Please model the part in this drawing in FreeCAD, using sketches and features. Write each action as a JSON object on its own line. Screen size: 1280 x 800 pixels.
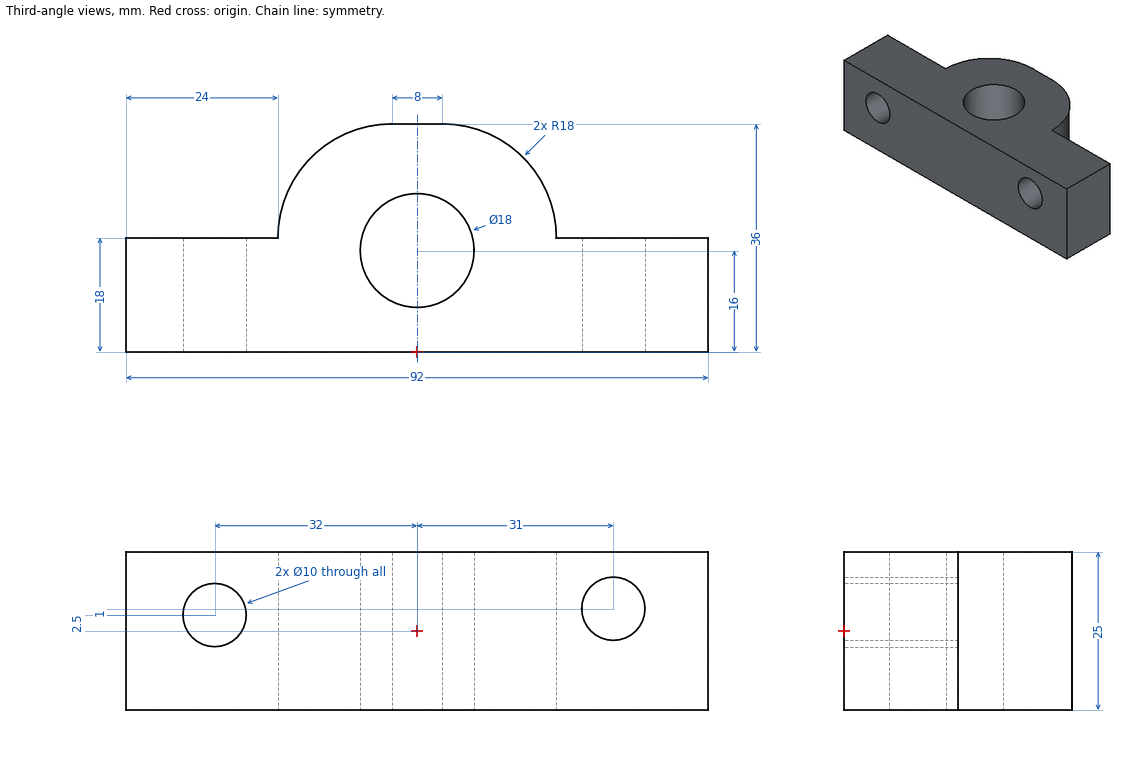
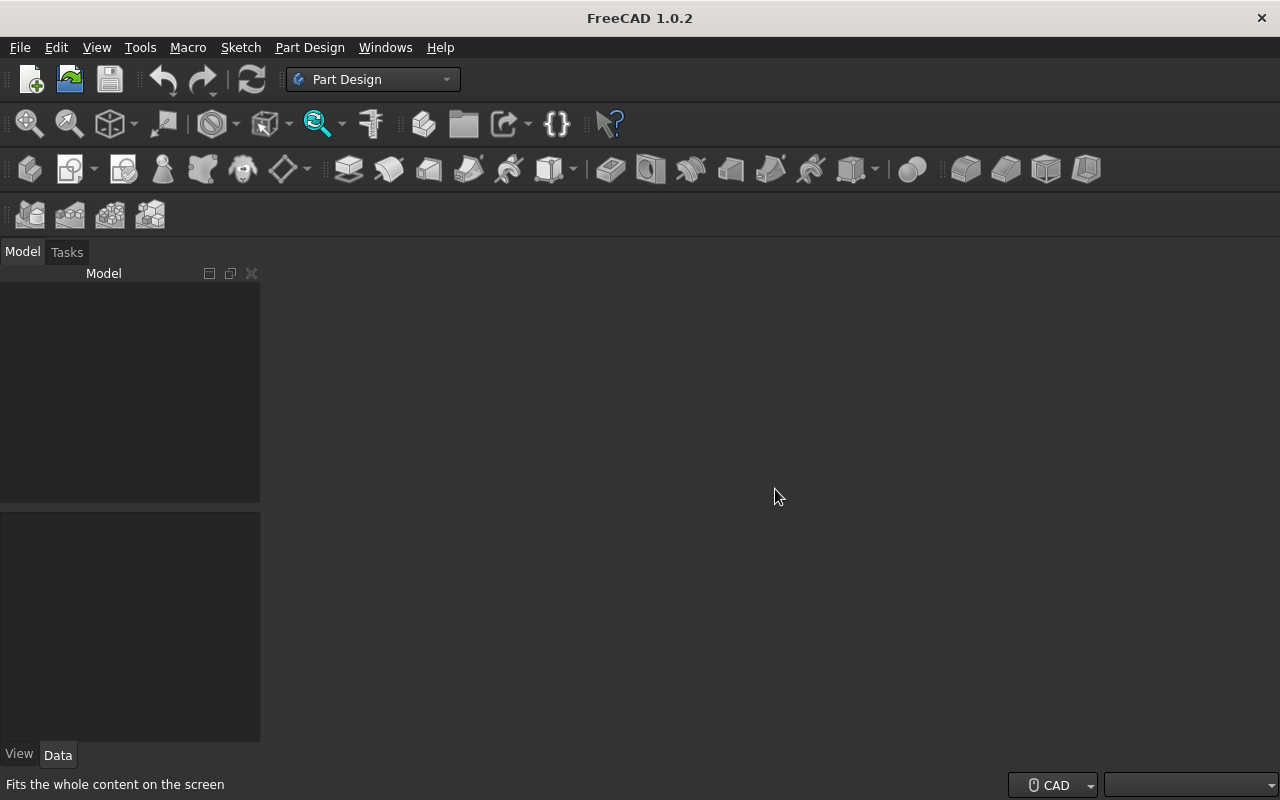
{"action": "left_click", "coordinate": [30, 80]}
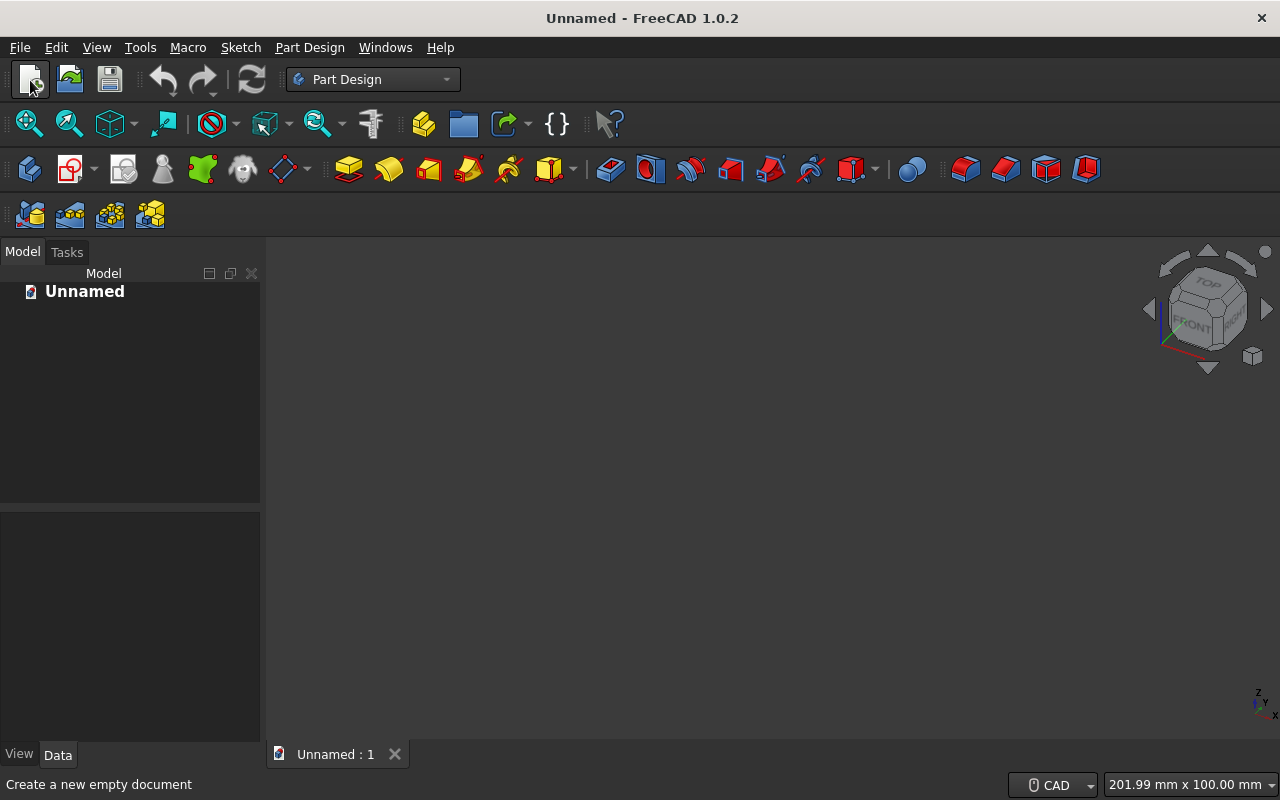
{"action": "left_click", "coordinate": [70, 170]}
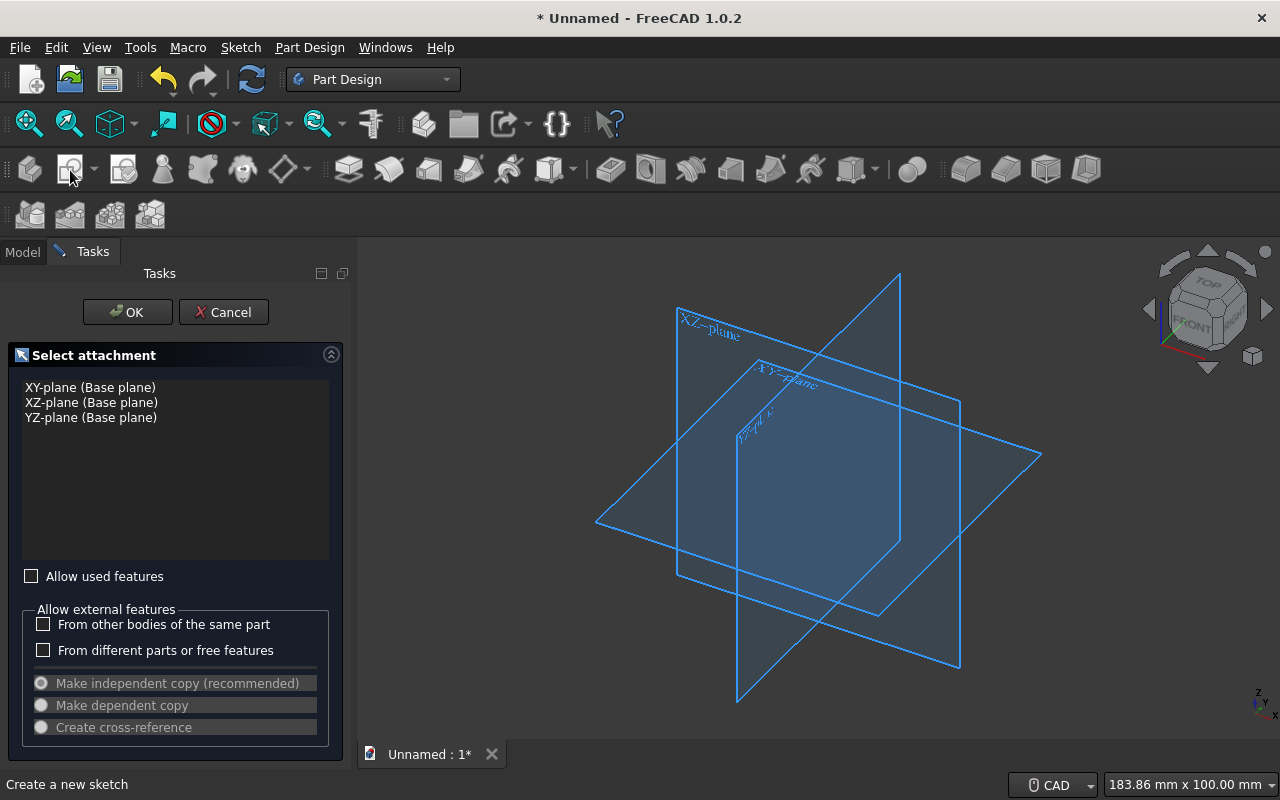
{"action": "left_click", "coordinate": [82, 388]}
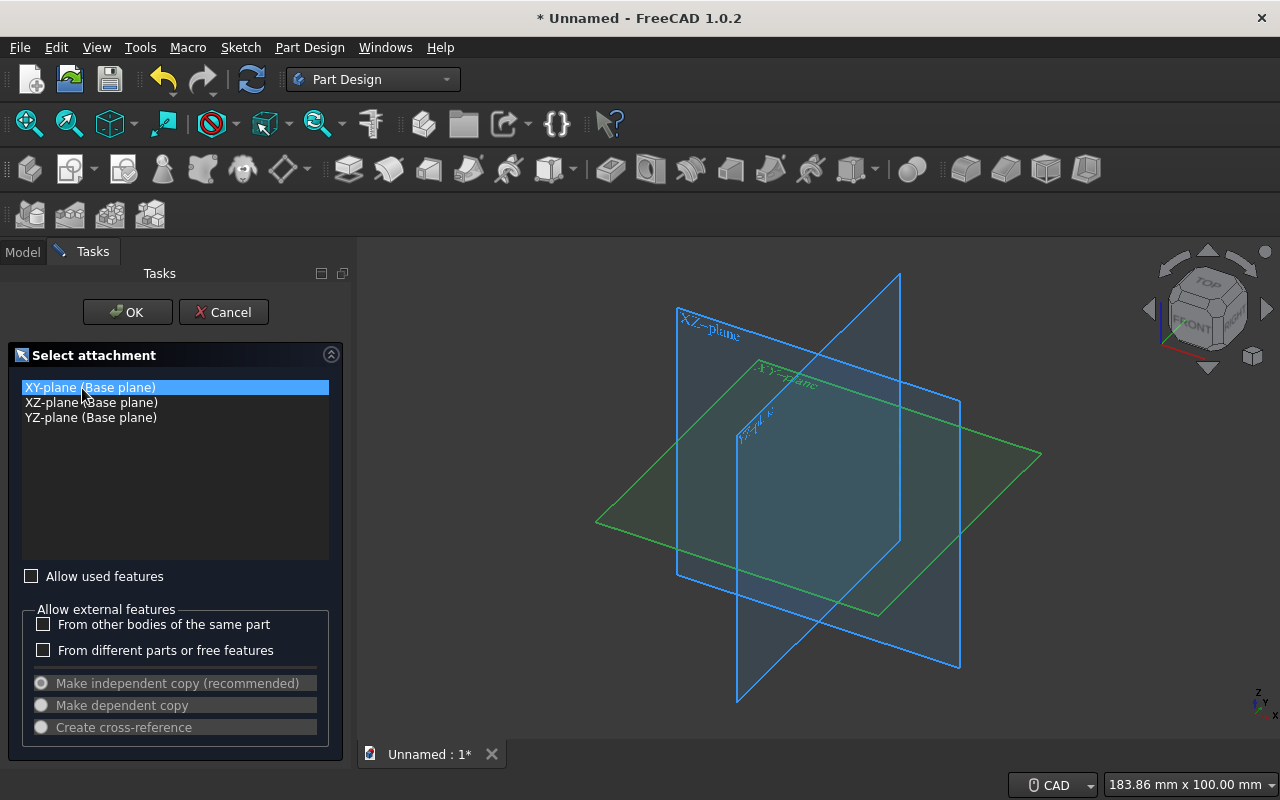
{"action": "left_click", "coordinate": [128, 312]}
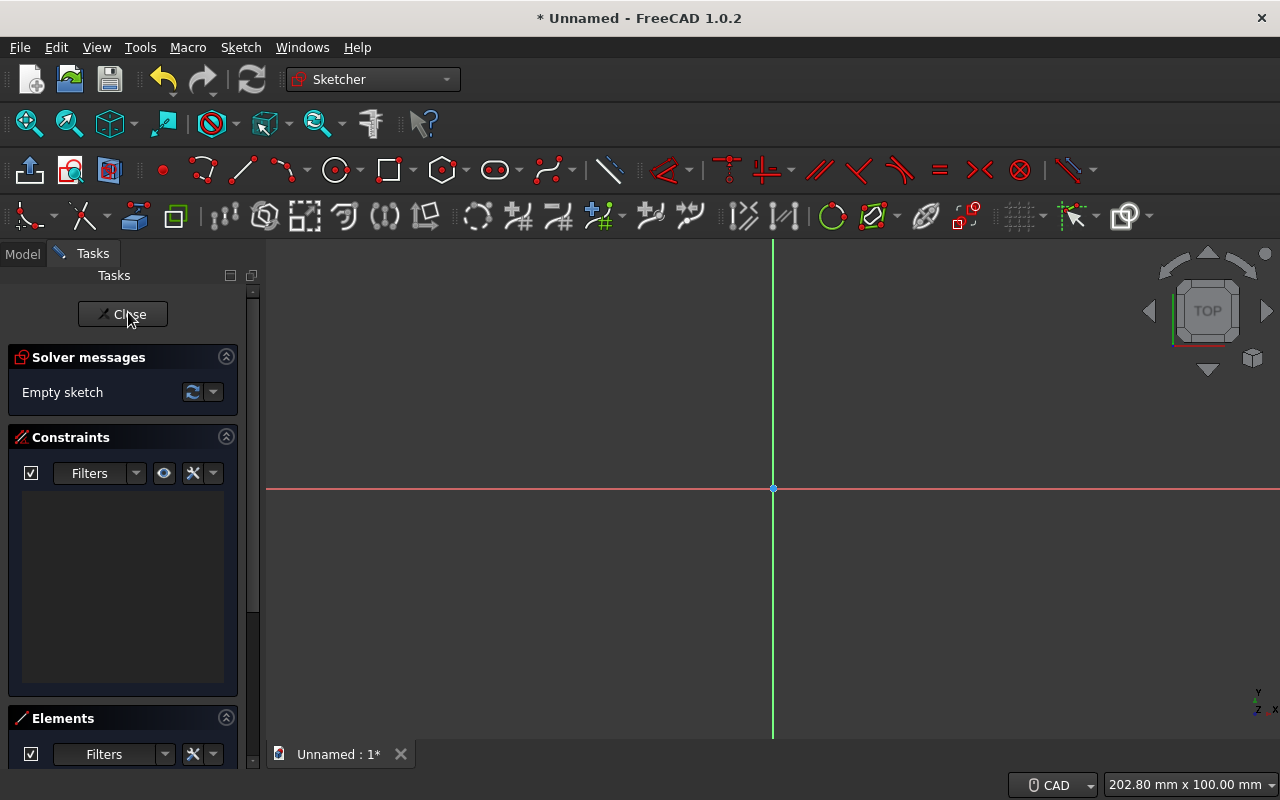
{"action": "key", "text": "g l"}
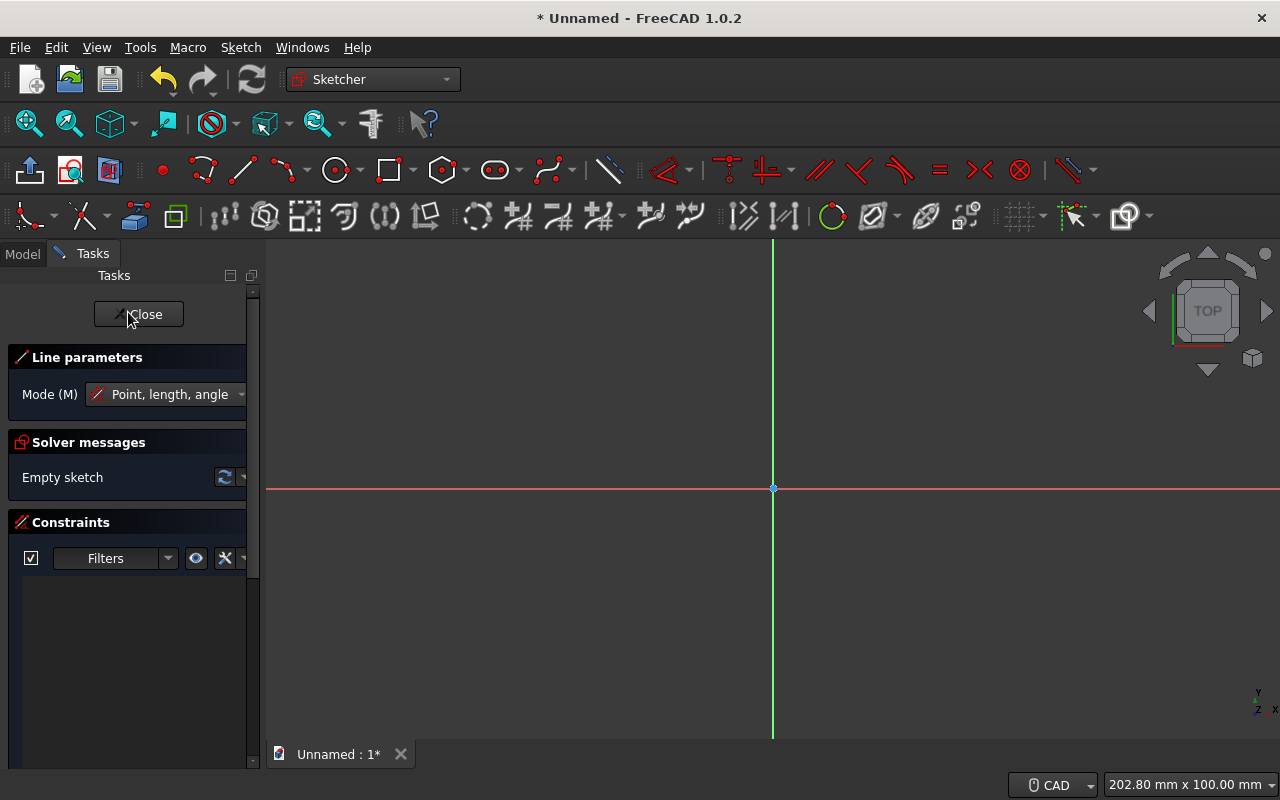
{"action": "left_click", "coordinate": [793, 309]}
{"action": "left_click", "coordinate": [753, 309]}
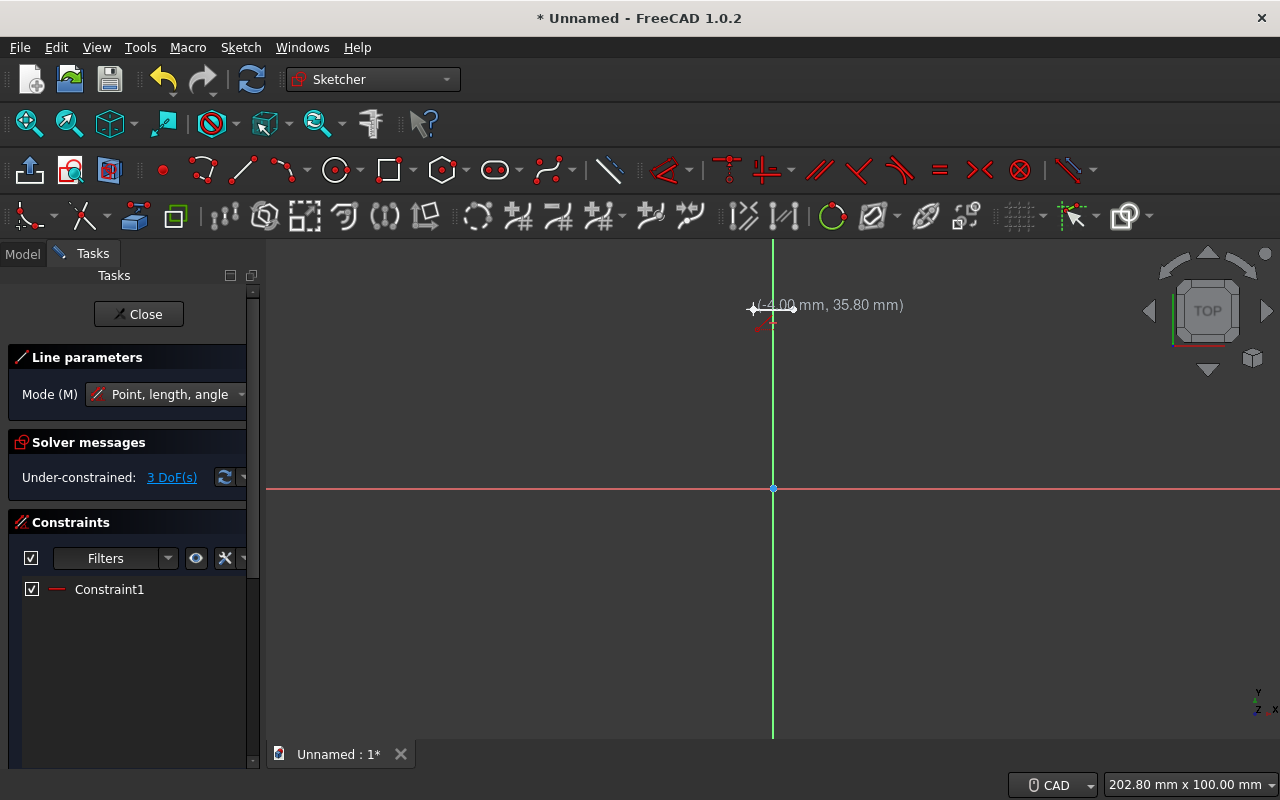
{"action": "left_click", "coordinate": [204, 170]}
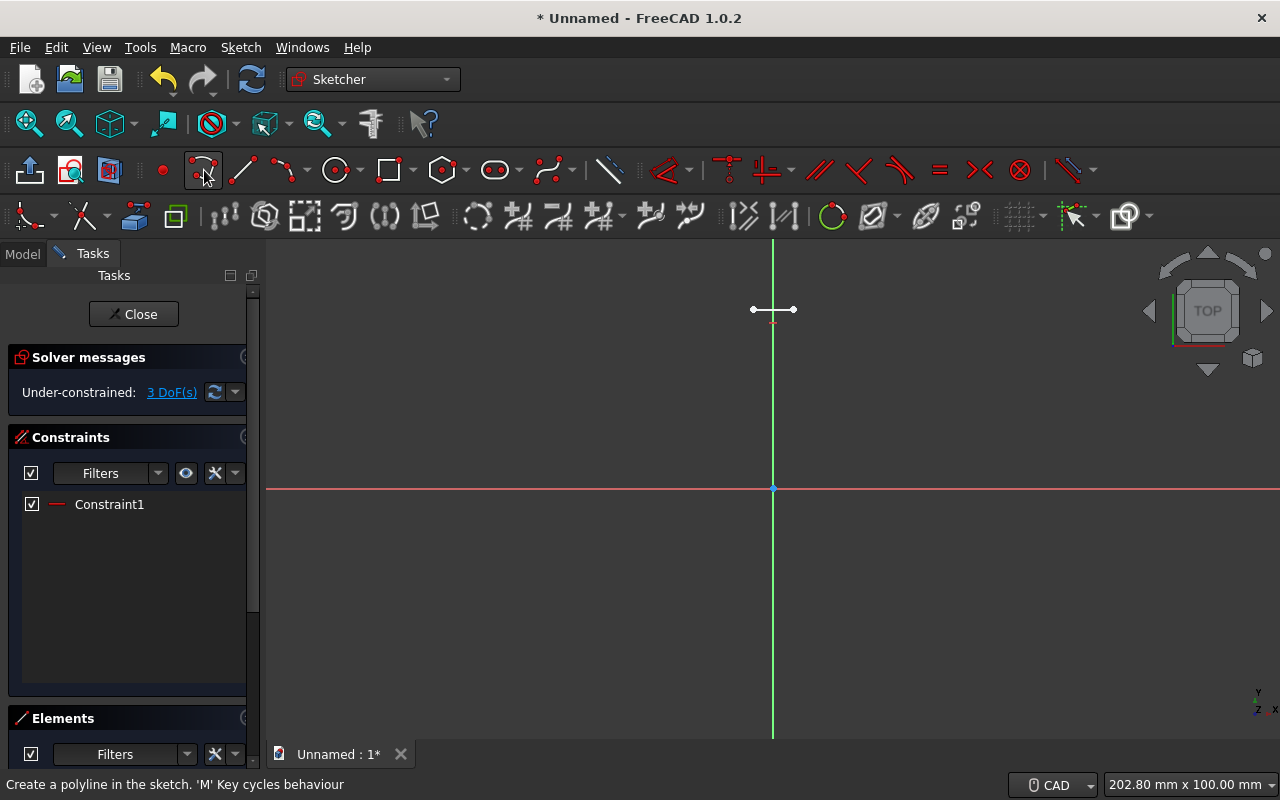
{"action": "left_click", "coordinate": [663, 399]}
{"action": "left_click", "coordinate": [543, 399]}
{"action": "left_click", "coordinate": [543, 489]}
{"action": "left_click", "coordinate": [1003, 480]}
{"action": "left_click", "coordinate": [1003, 399]}
{"action": "left_click", "coordinate": [883, 399]}
{"action": "right_click", "coordinate": [883, 399]}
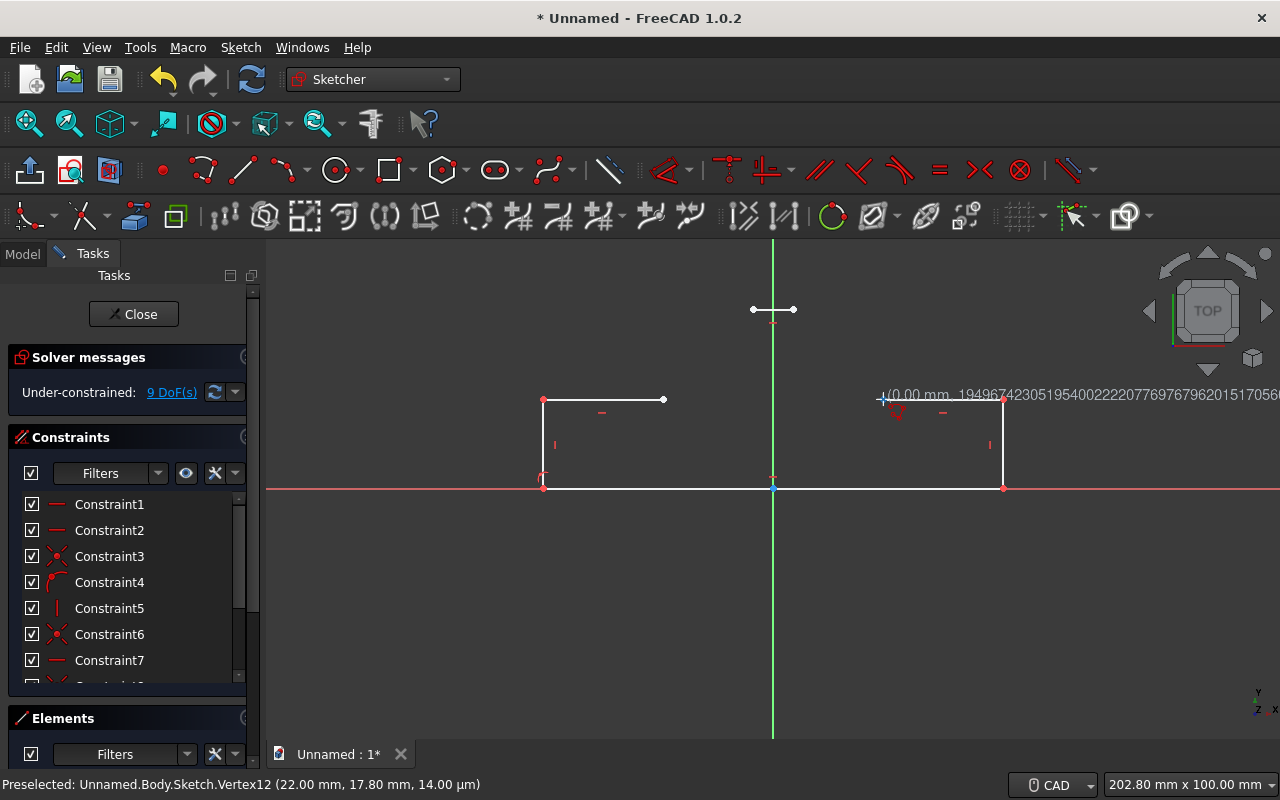
{"action": "left_click", "coordinate": [284, 170]}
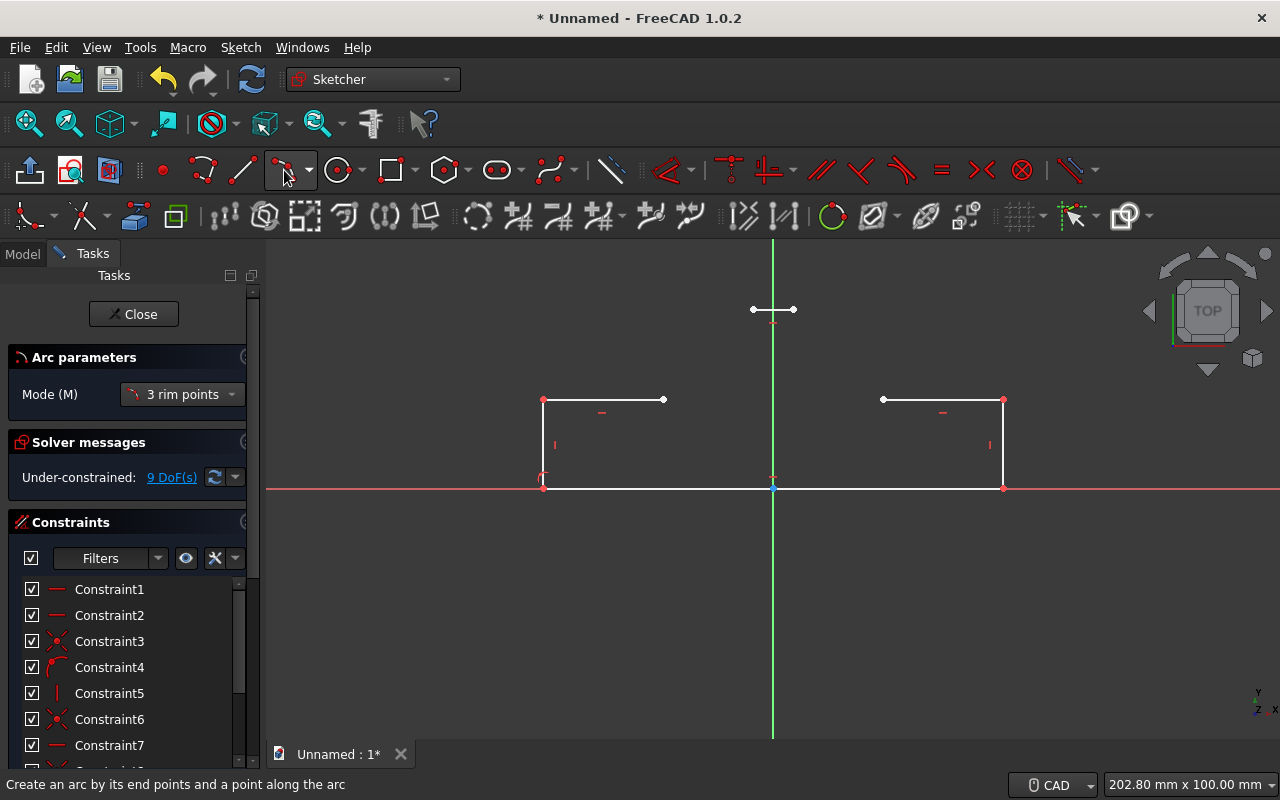
{"action": "left_click", "coordinate": [753, 310]}
{"action": "left_click", "coordinate": [663, 400]}
{"action": "left_click", "coordinate": [689, 335]}